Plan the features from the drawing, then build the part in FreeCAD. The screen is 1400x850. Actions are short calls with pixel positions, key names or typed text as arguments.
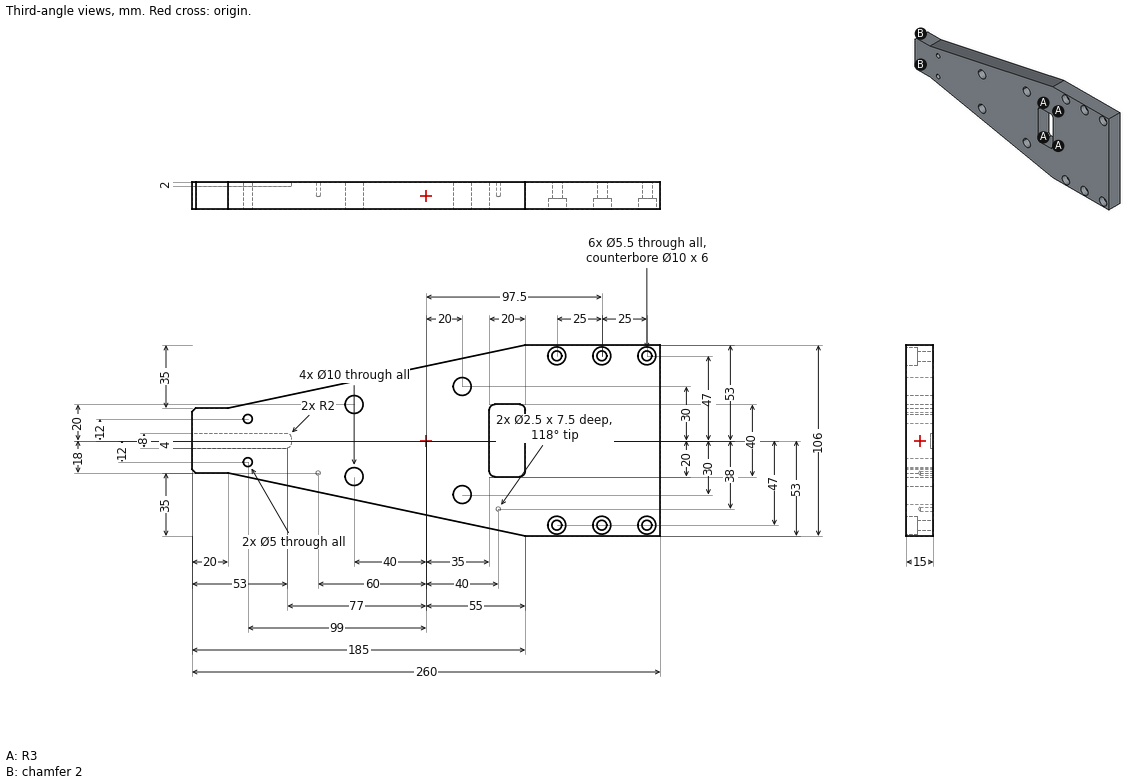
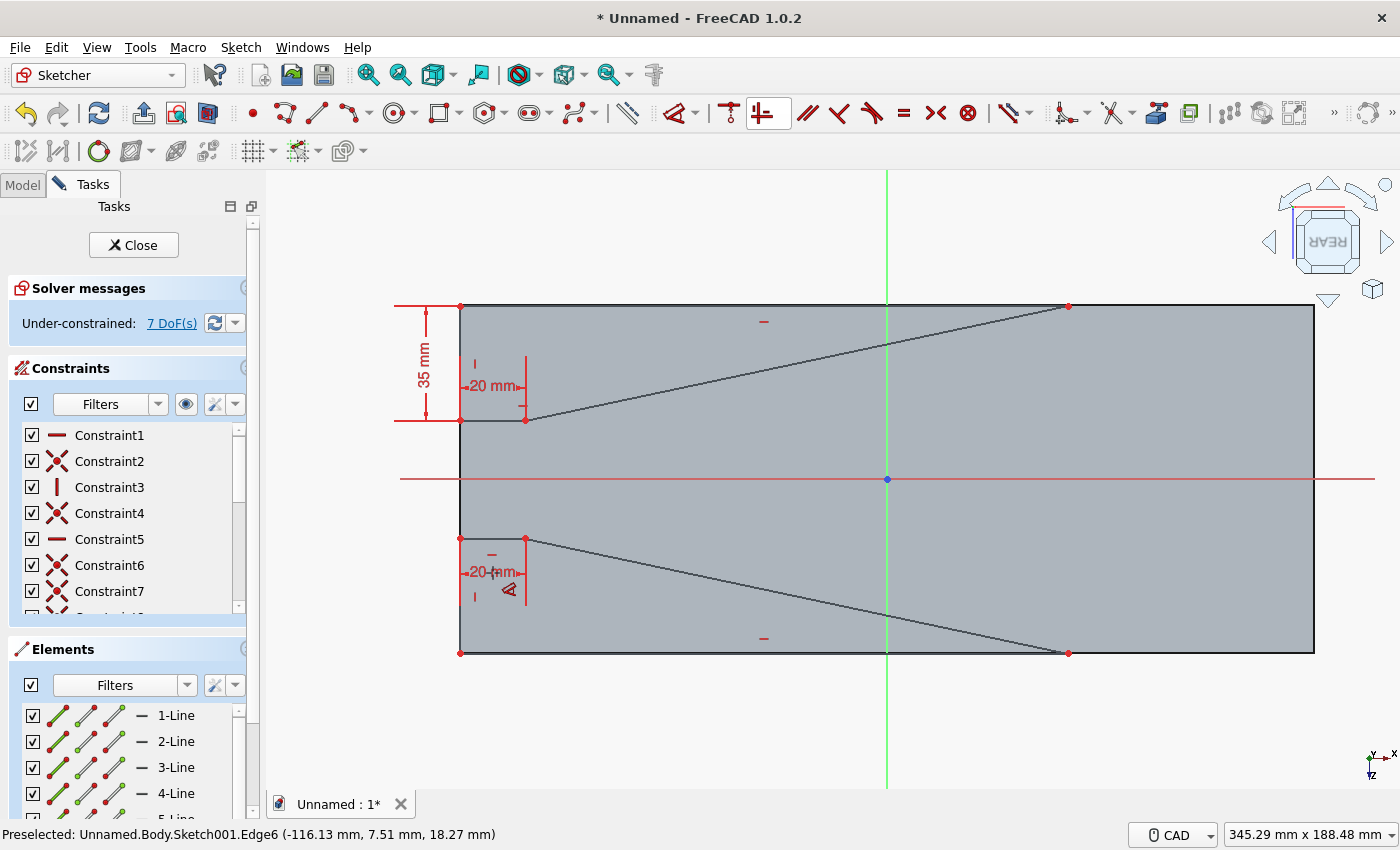
click(460, 573)
click(426, 596)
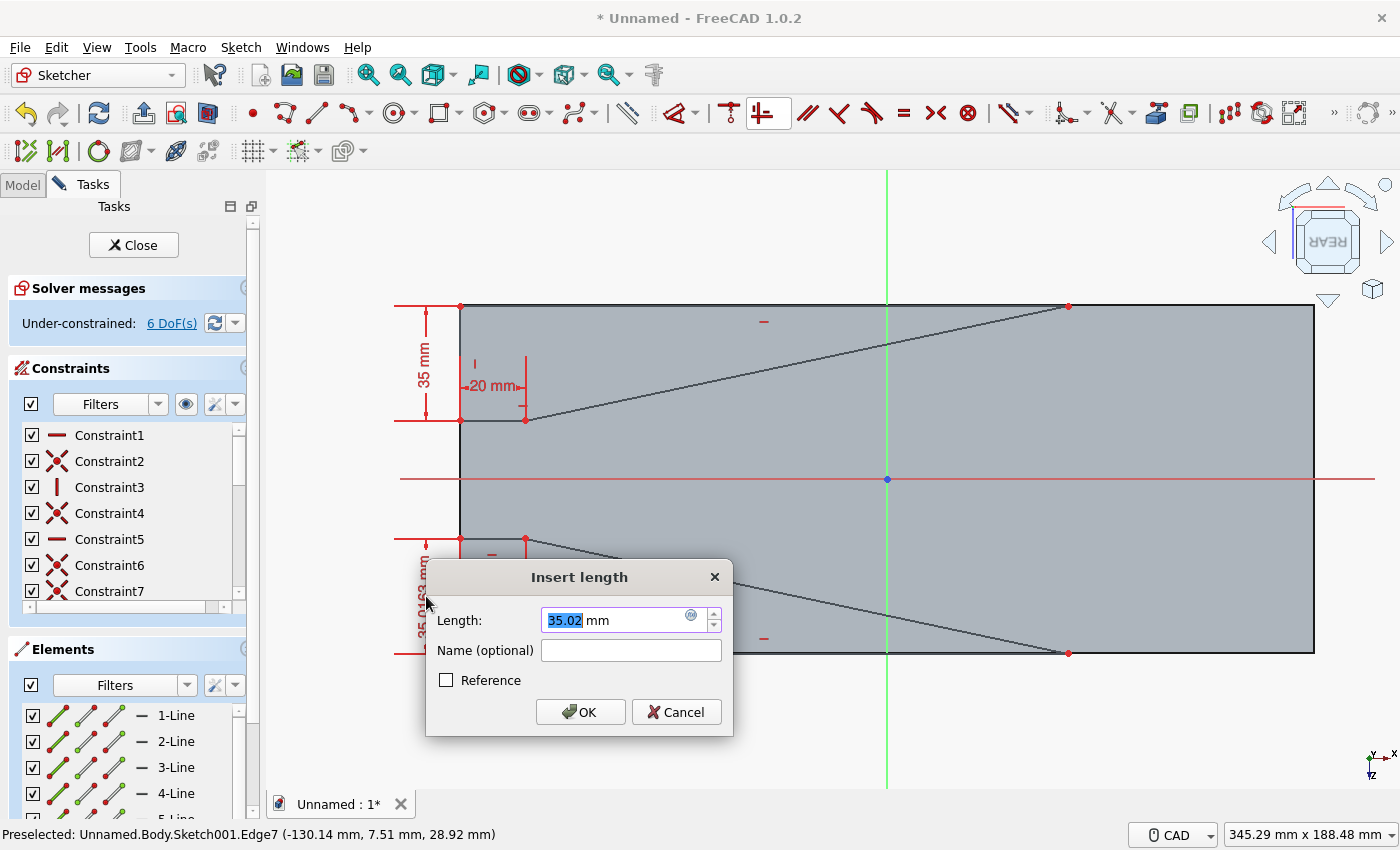
text(35)
key(Return)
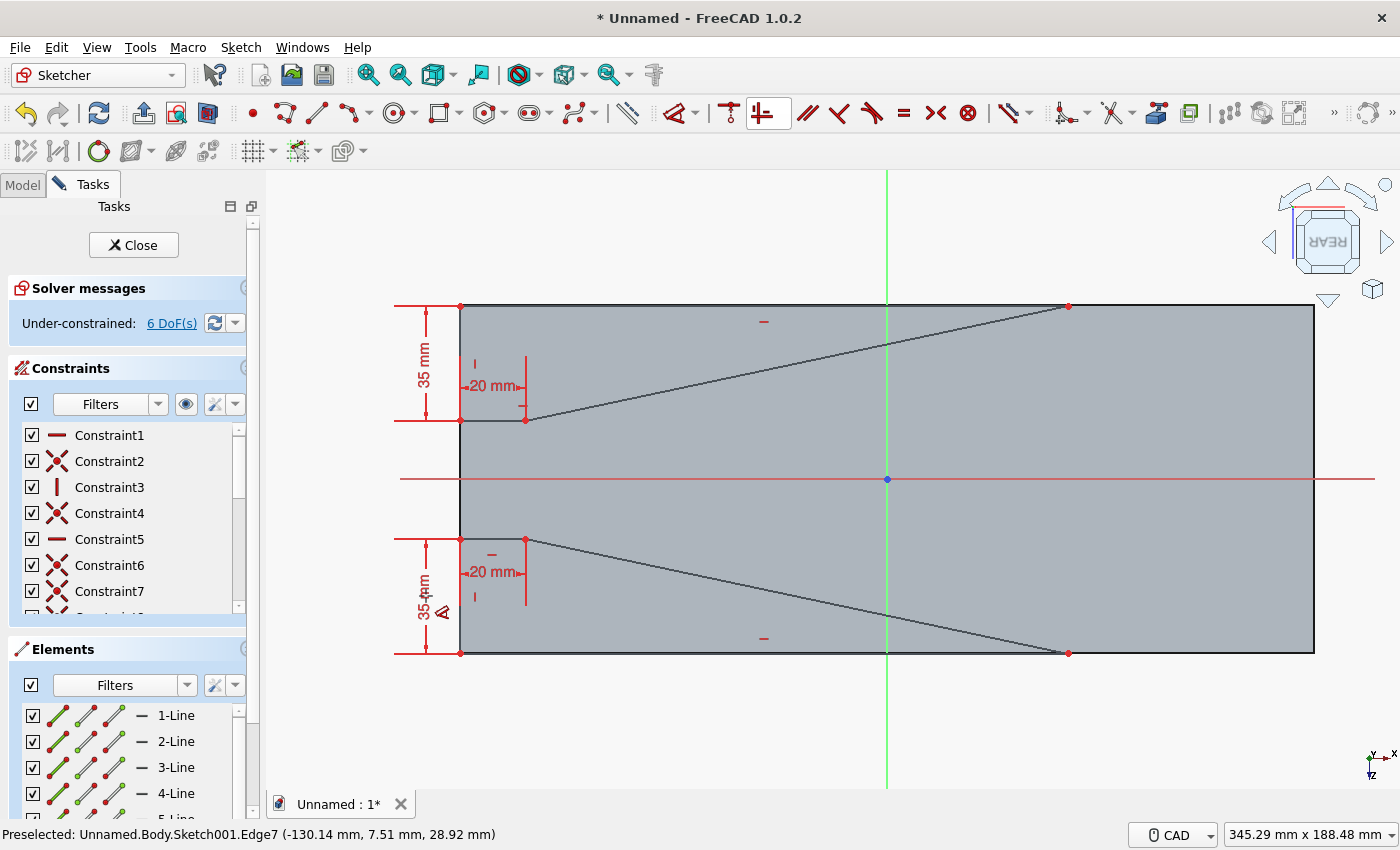
click(886, 306)
click(764, 272)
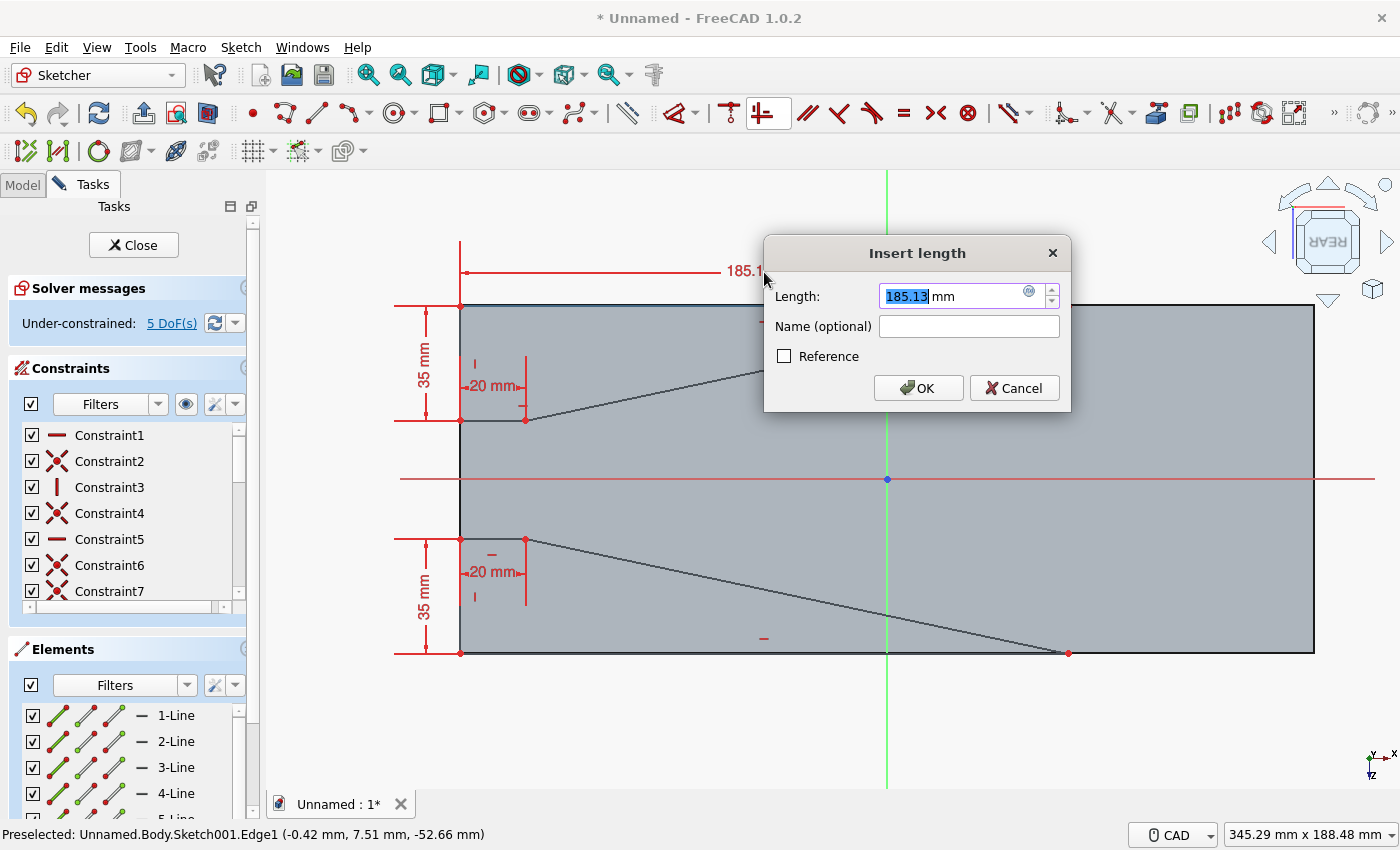
text(185)
key(Return)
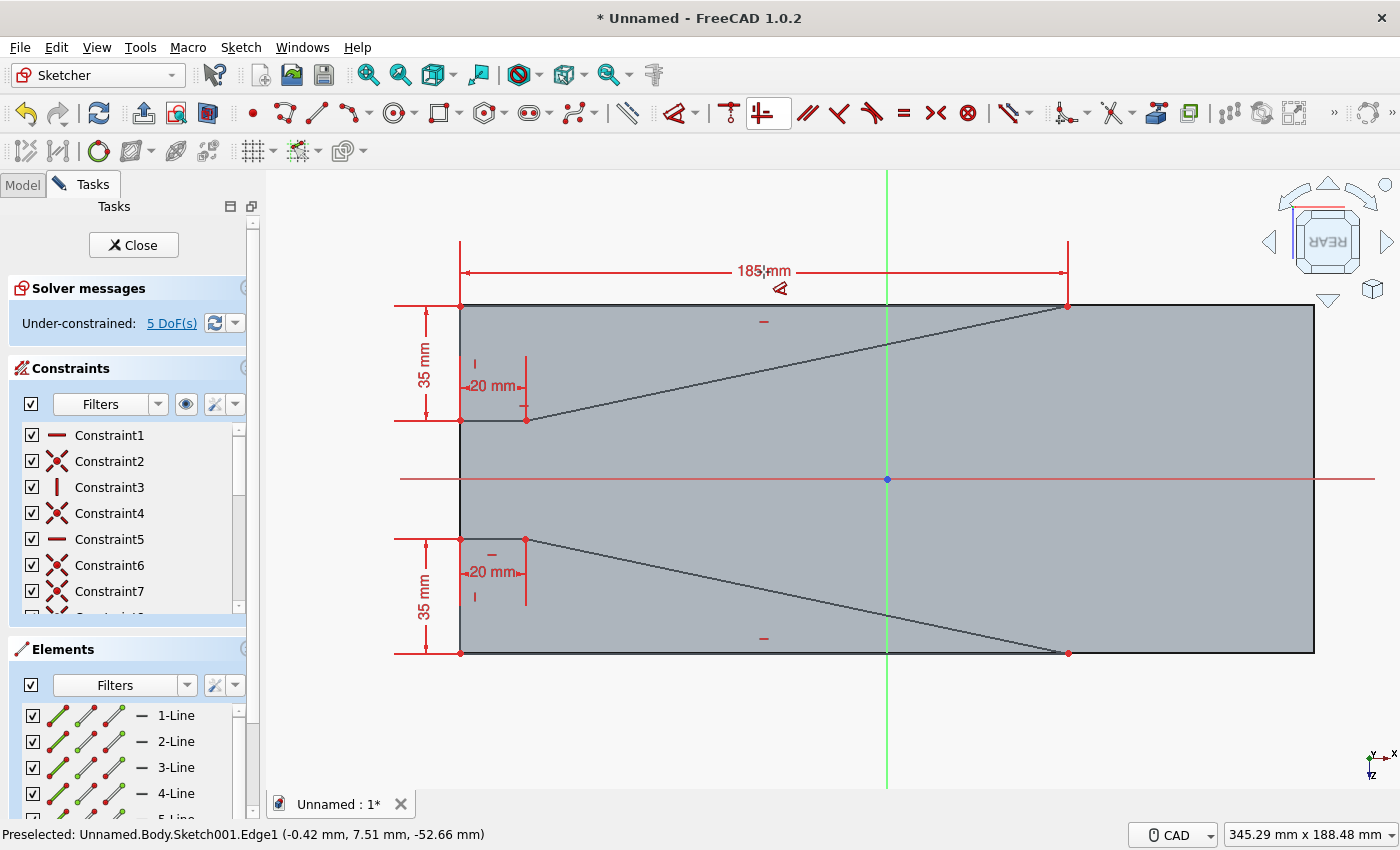
click(642, 654)
click(764, 688)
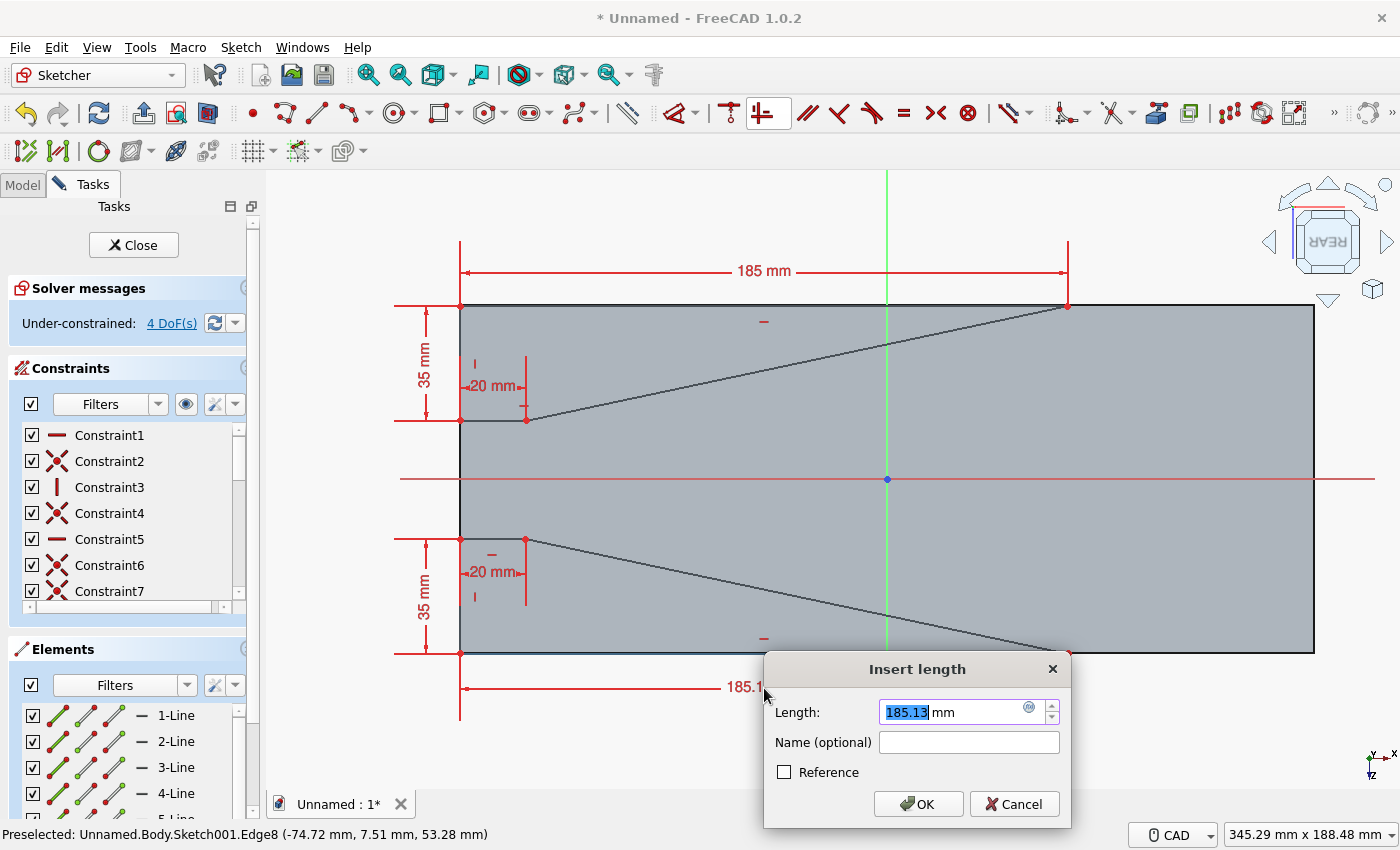
text(185)
key(Return)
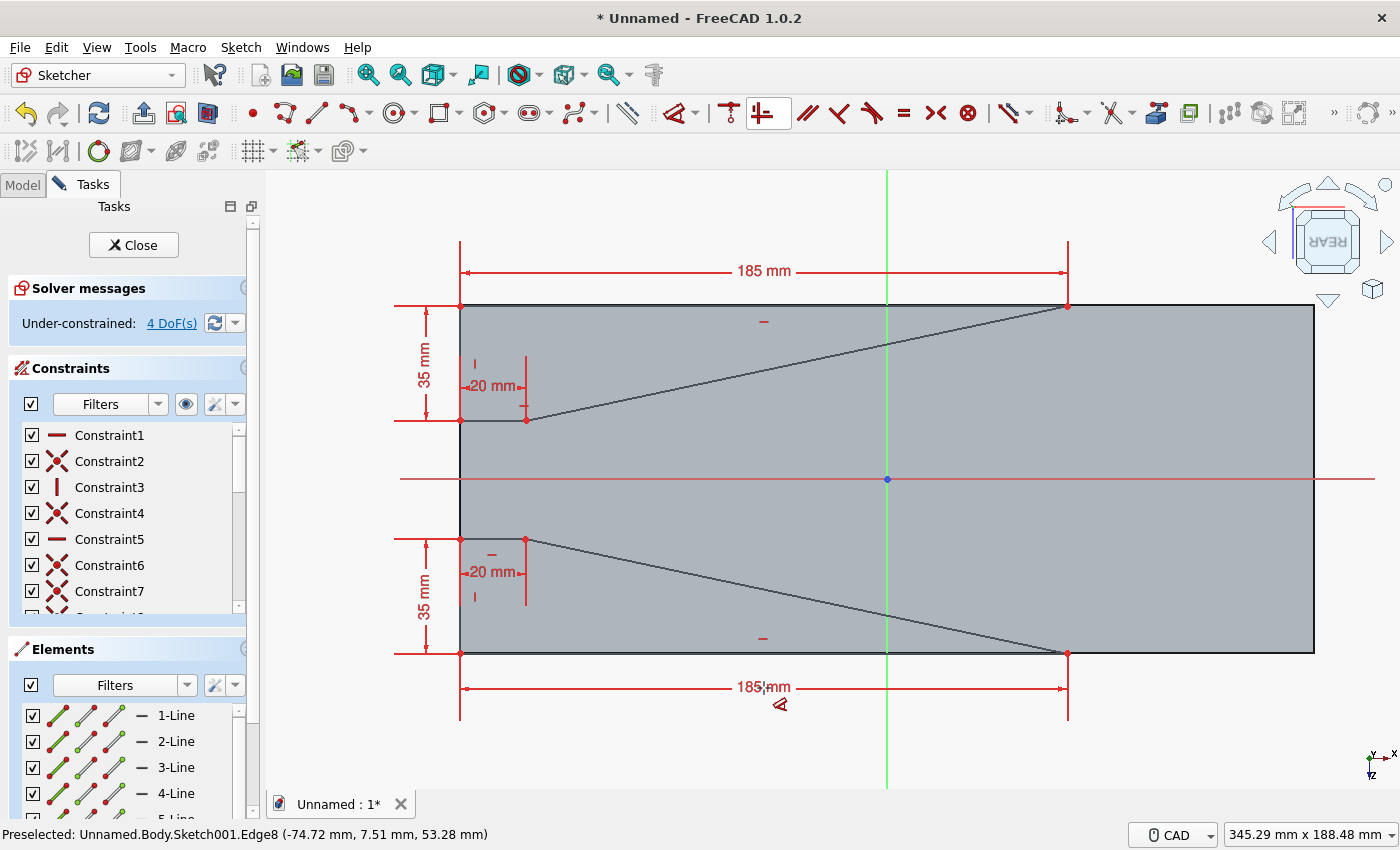
click(1068, 306)
click(978, 272)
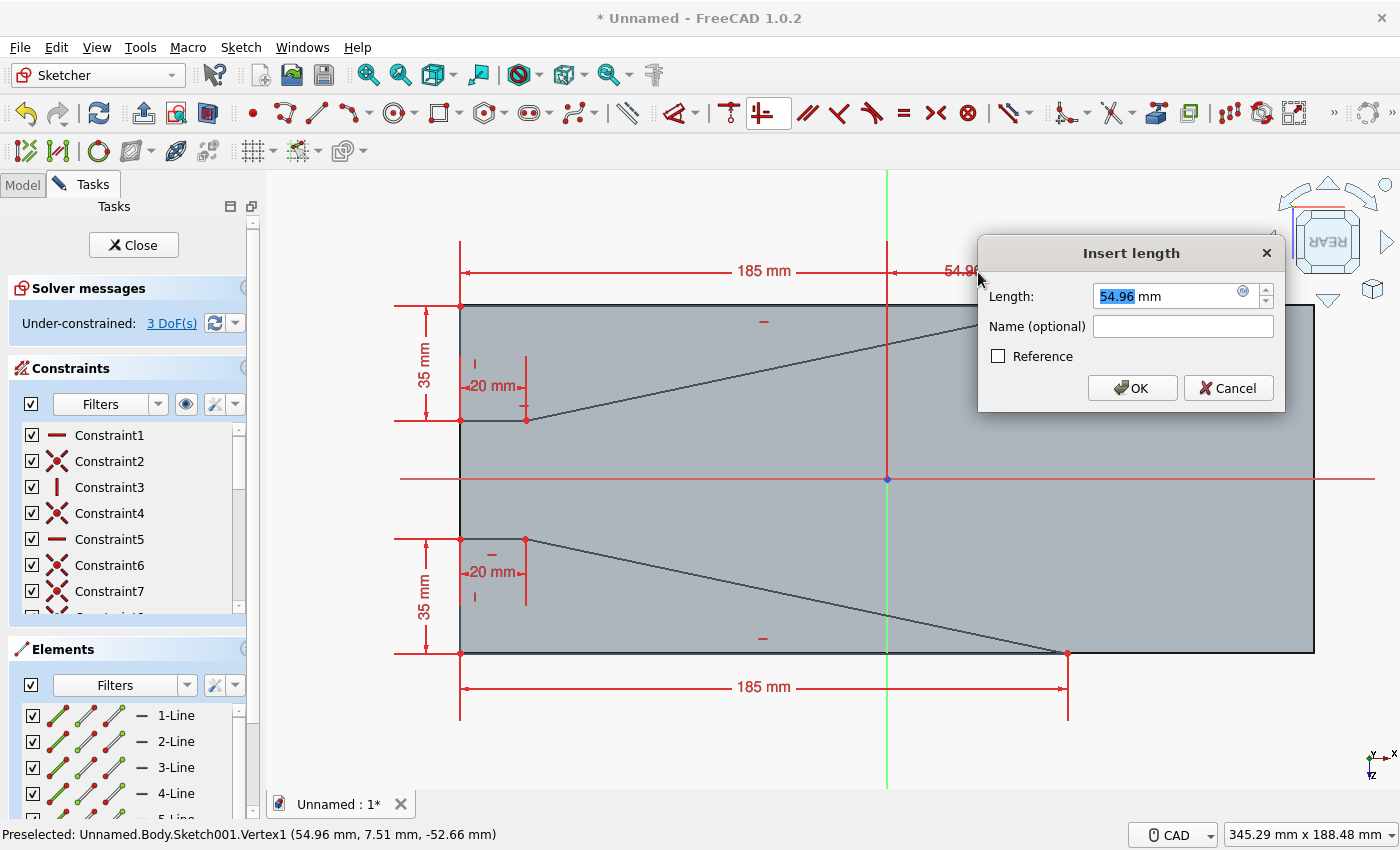
text(55)
key(Return)